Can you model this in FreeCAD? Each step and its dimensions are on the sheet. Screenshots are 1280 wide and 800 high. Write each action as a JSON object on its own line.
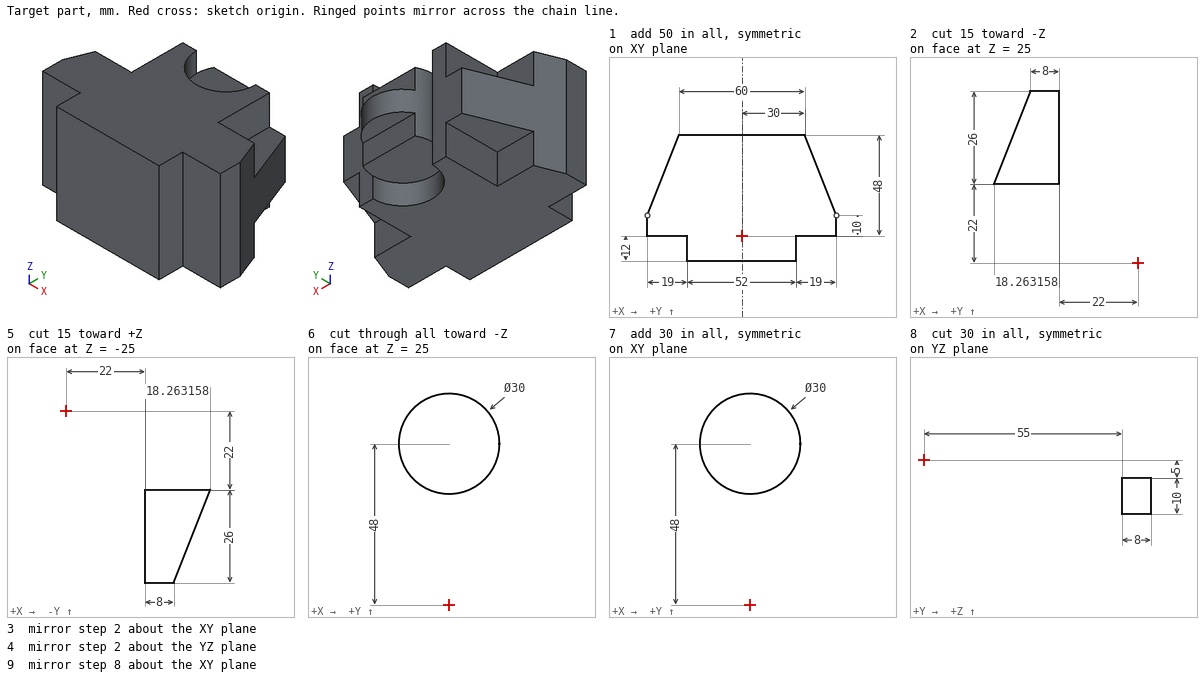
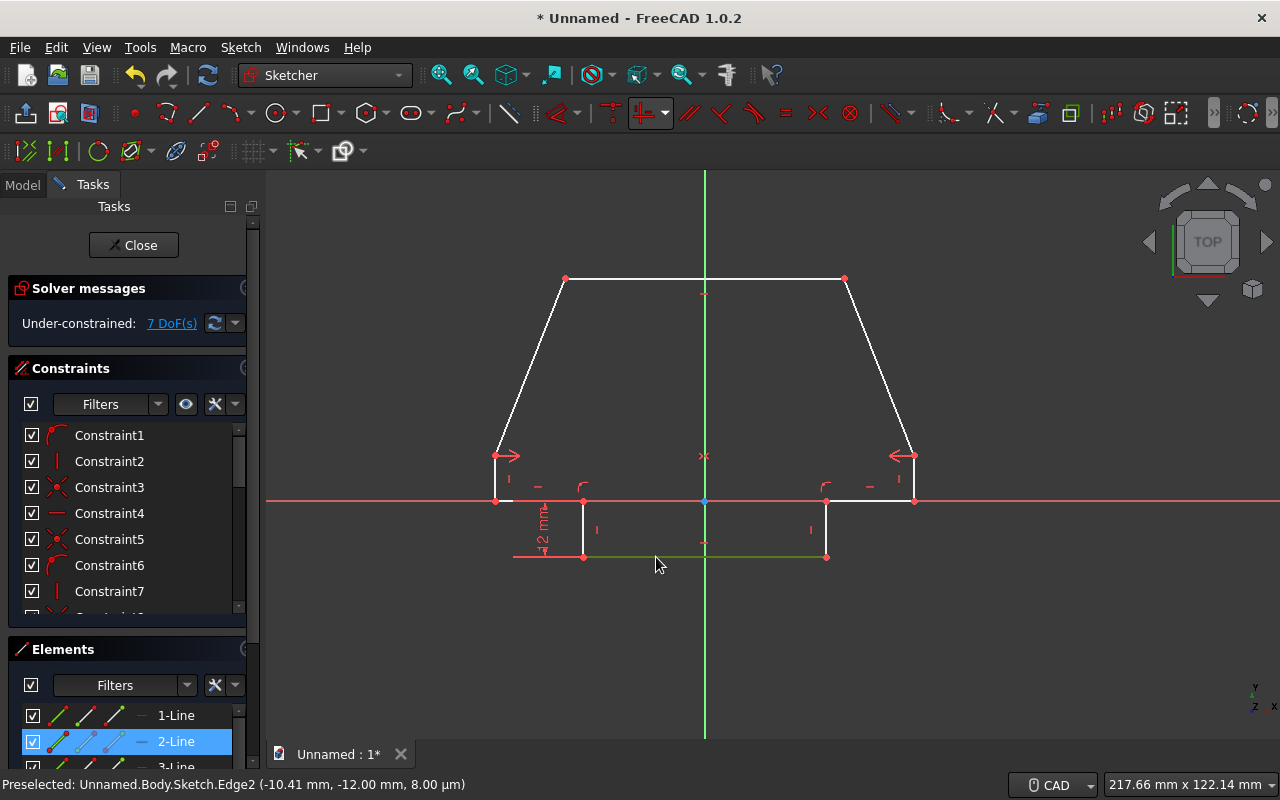
{"action": "key", "text": "l"}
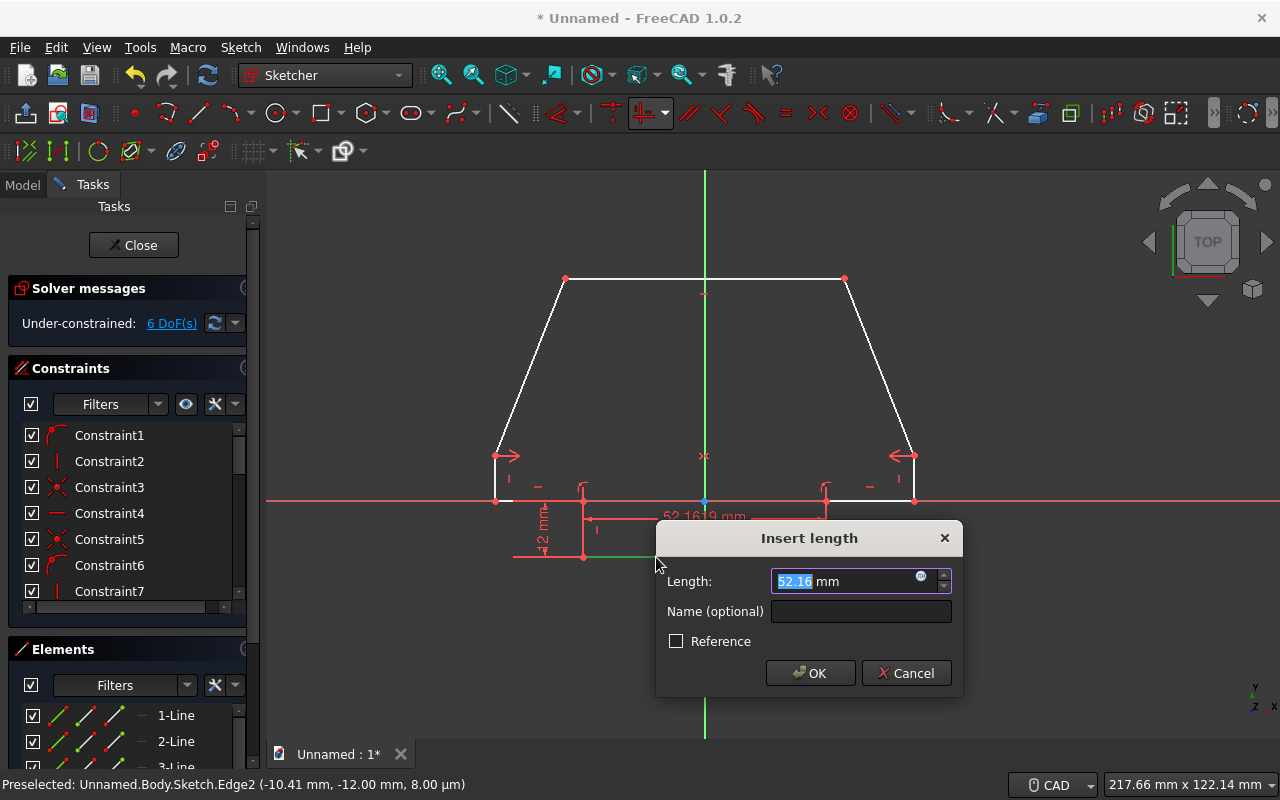
{"action": "type", "text": "52"}
{"action": "key", "text": "Return"}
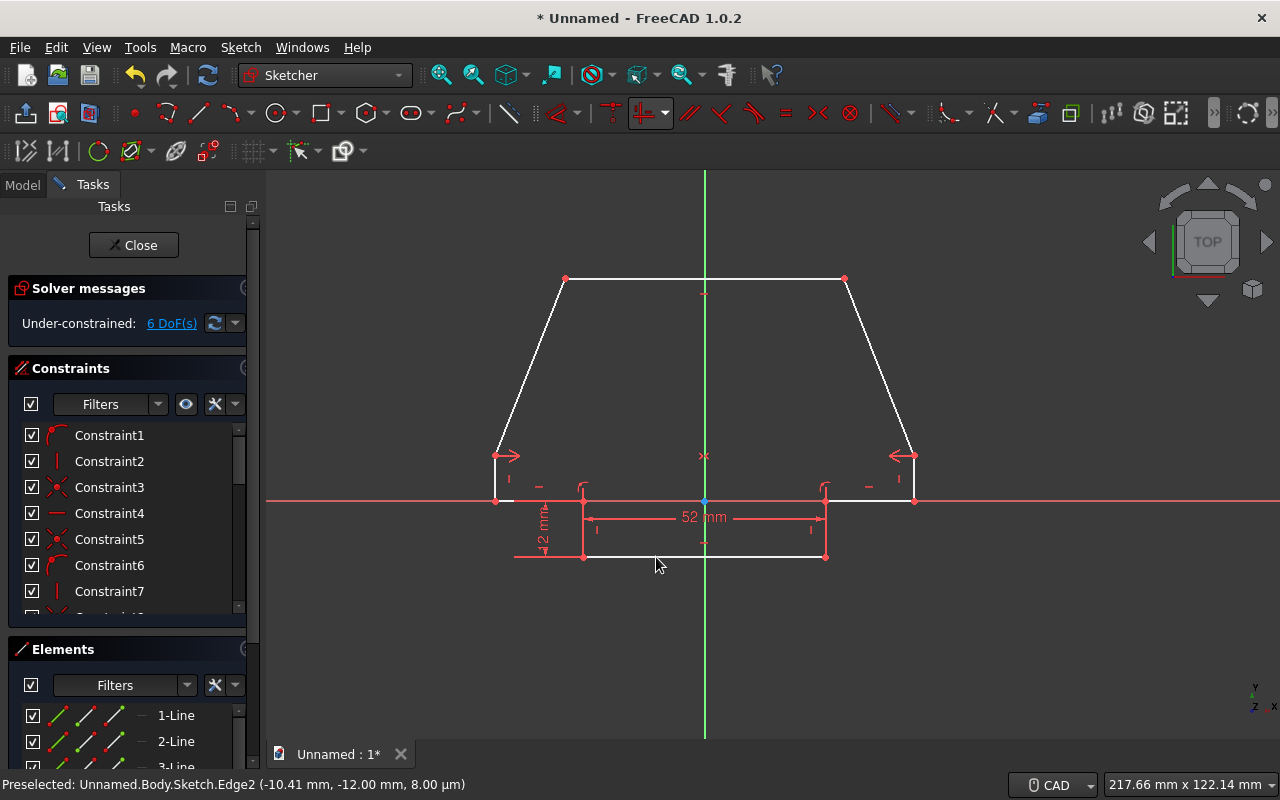
{"action": "left_click", "coordinate": [852, 501]}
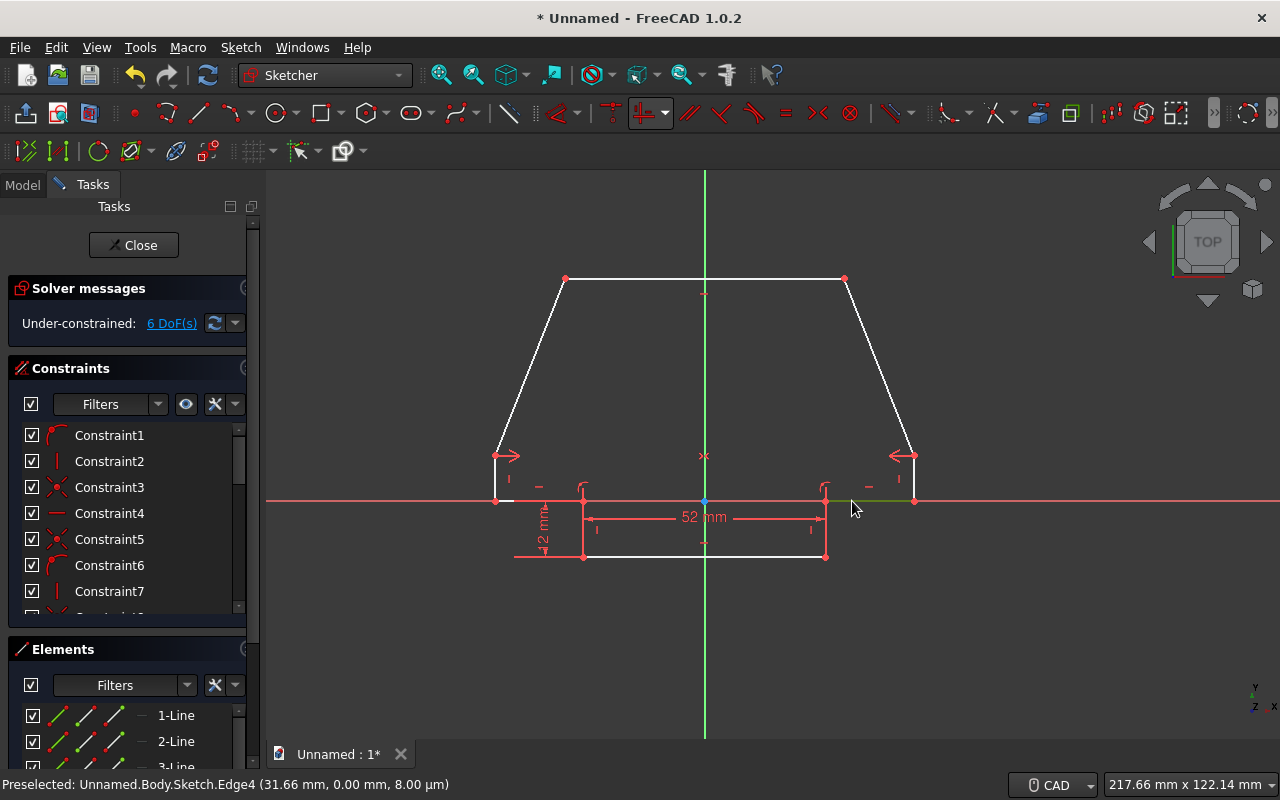
{"action": "key", "text": "l"}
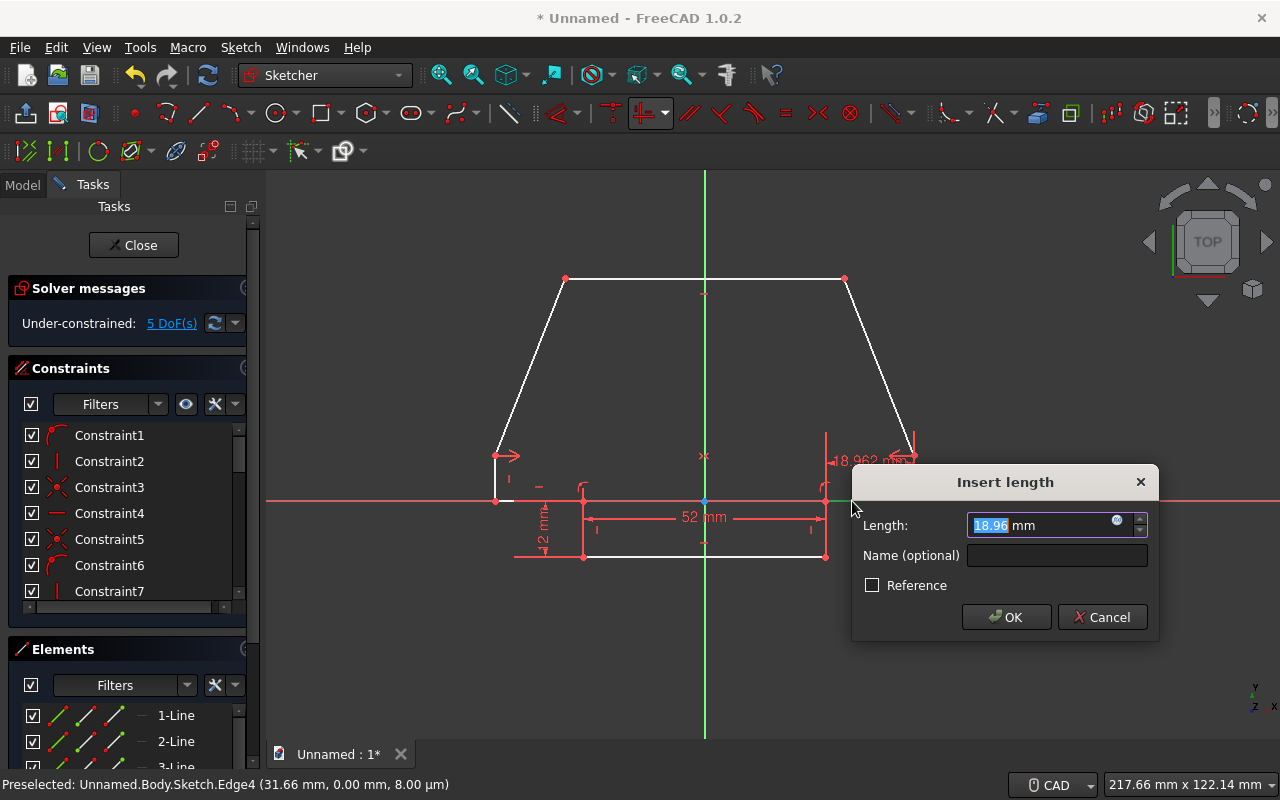
{"action": "type", "text": "19"}
{"action": "key", "text": "Return"}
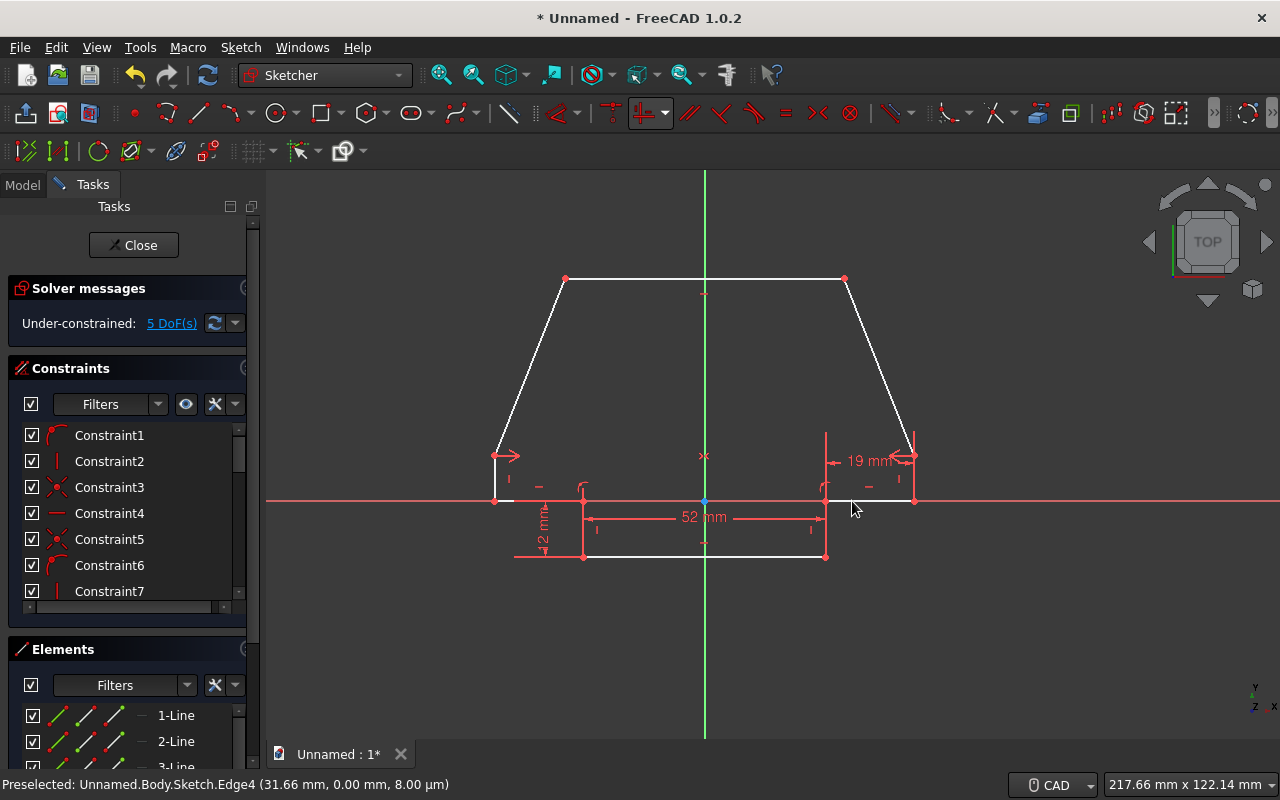
{"action": "left_click", "coordinate": [914, 488]}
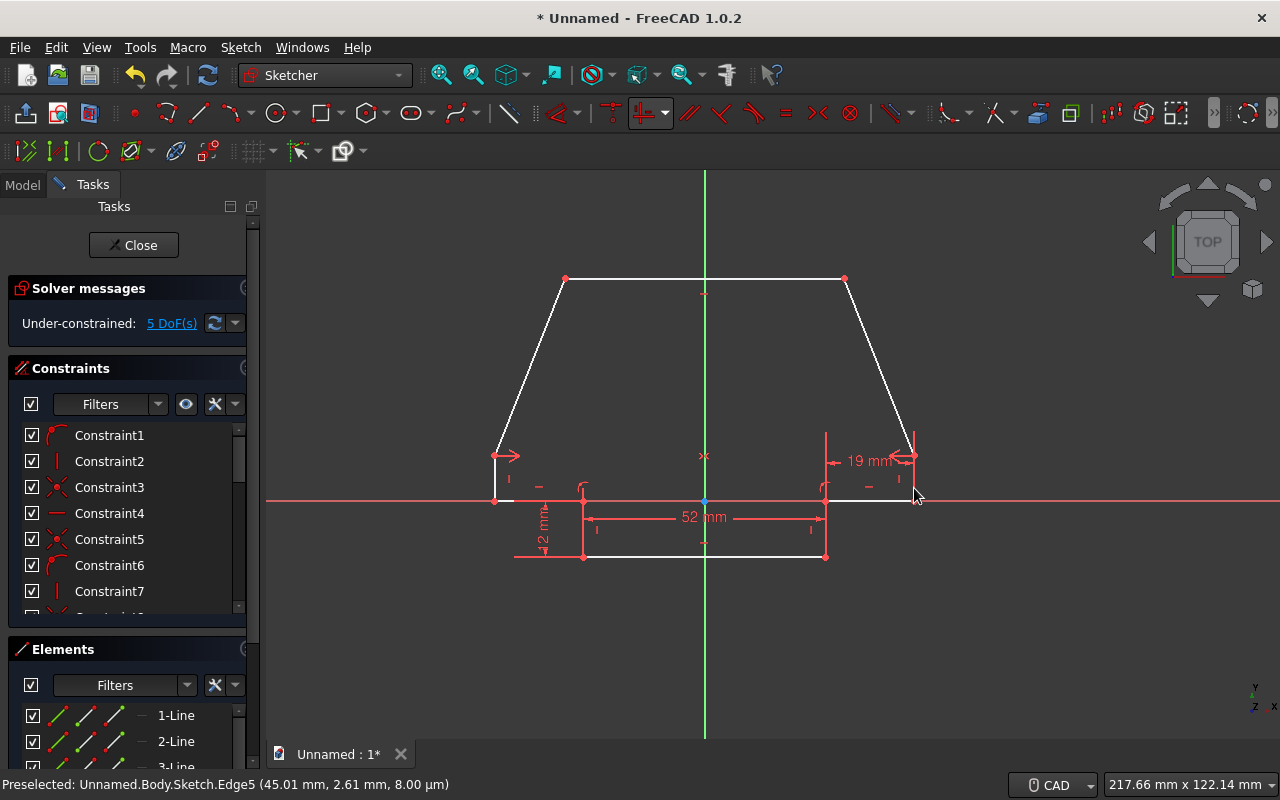
{"action": "left_click", "coordinate": [580, 114]}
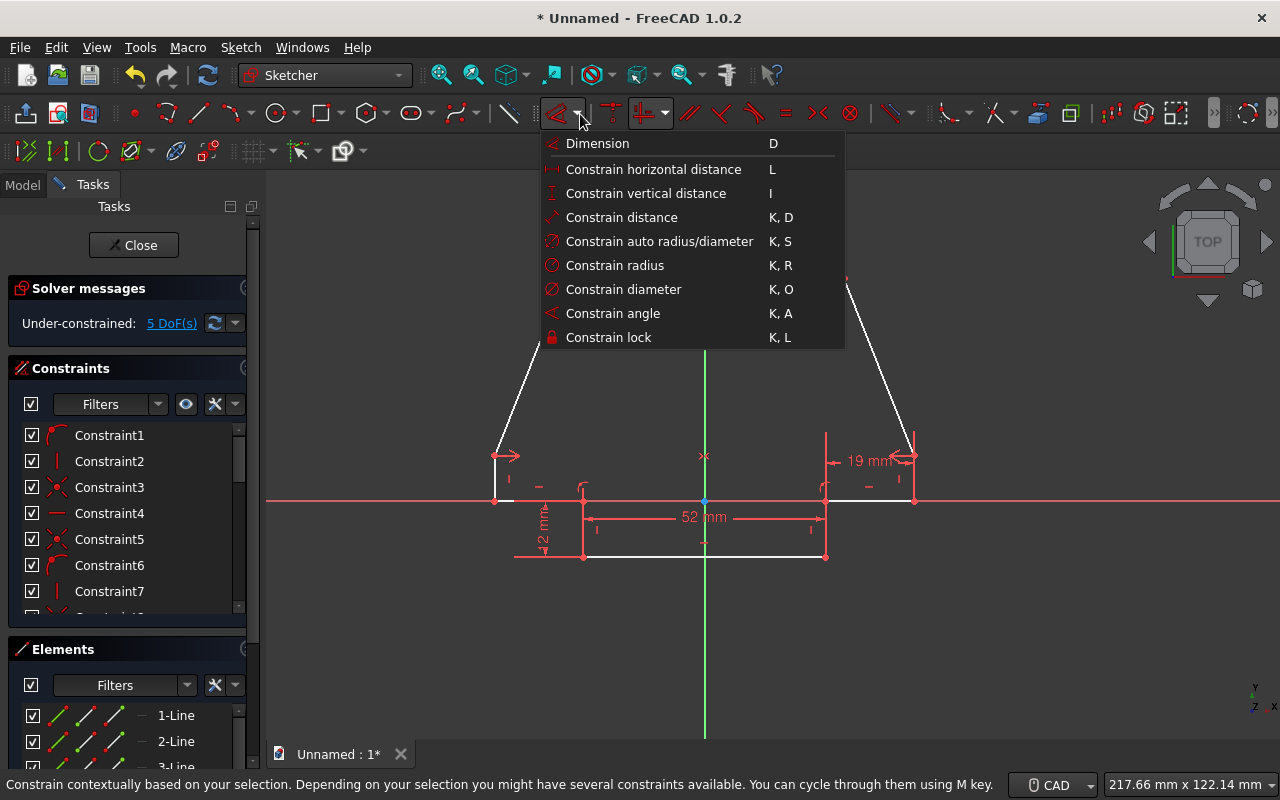
{"action": "left_click", "coordinate": [693, 193]}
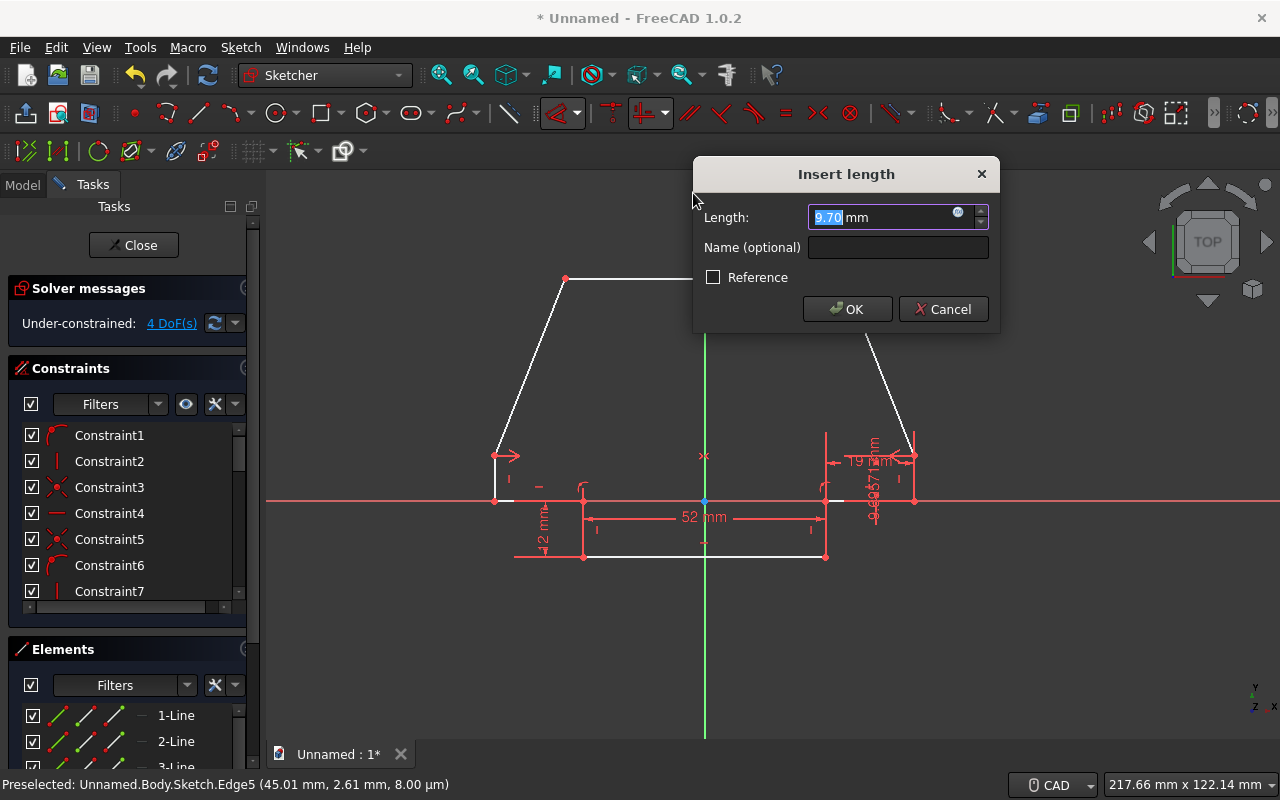
{"action": "type", "text": "10"}
{"action": "key", "text": "Return"}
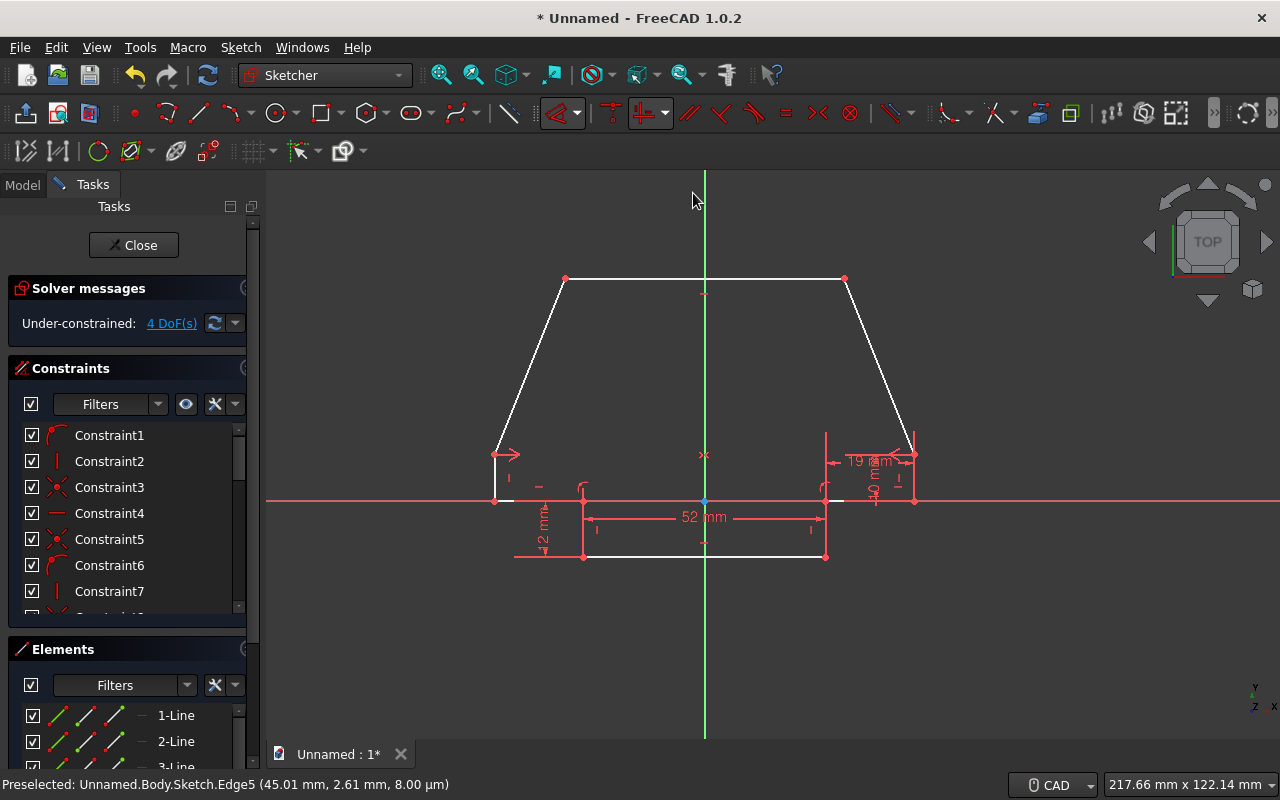
{"action": "left_click", "coordinate": [760, 279]}